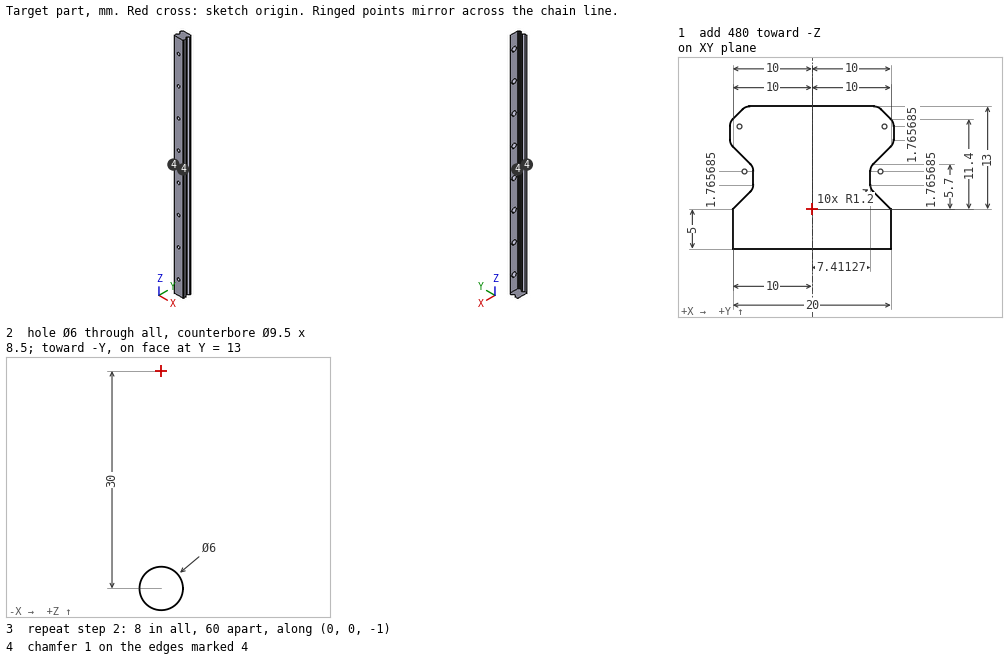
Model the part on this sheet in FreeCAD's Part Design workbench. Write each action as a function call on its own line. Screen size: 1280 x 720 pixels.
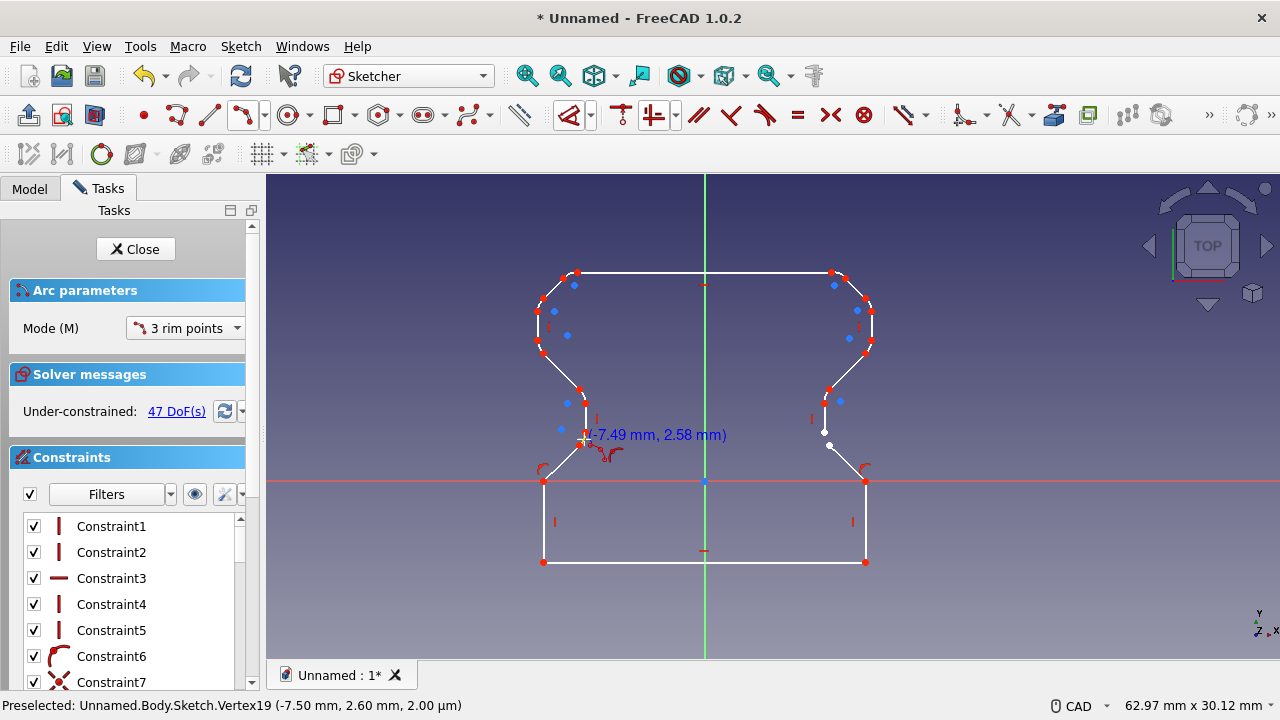
click(830, 446)
click(825, 433)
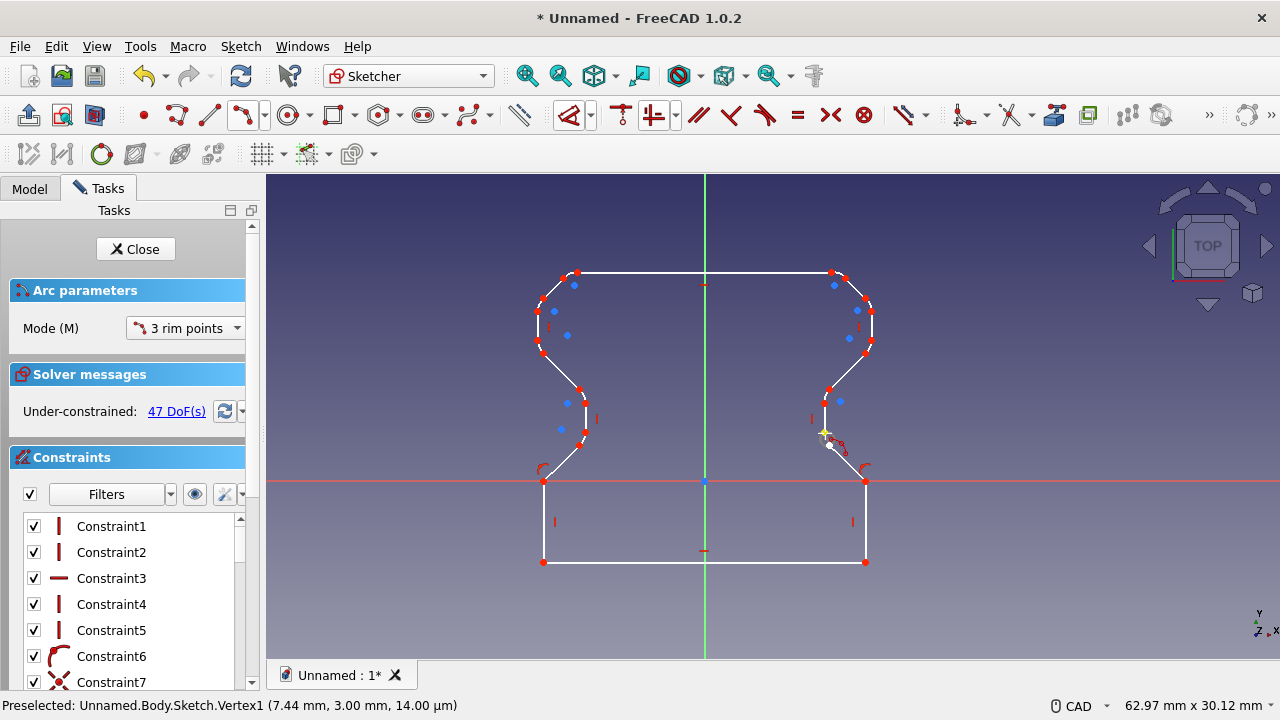
scroll(826, 439, up, 12)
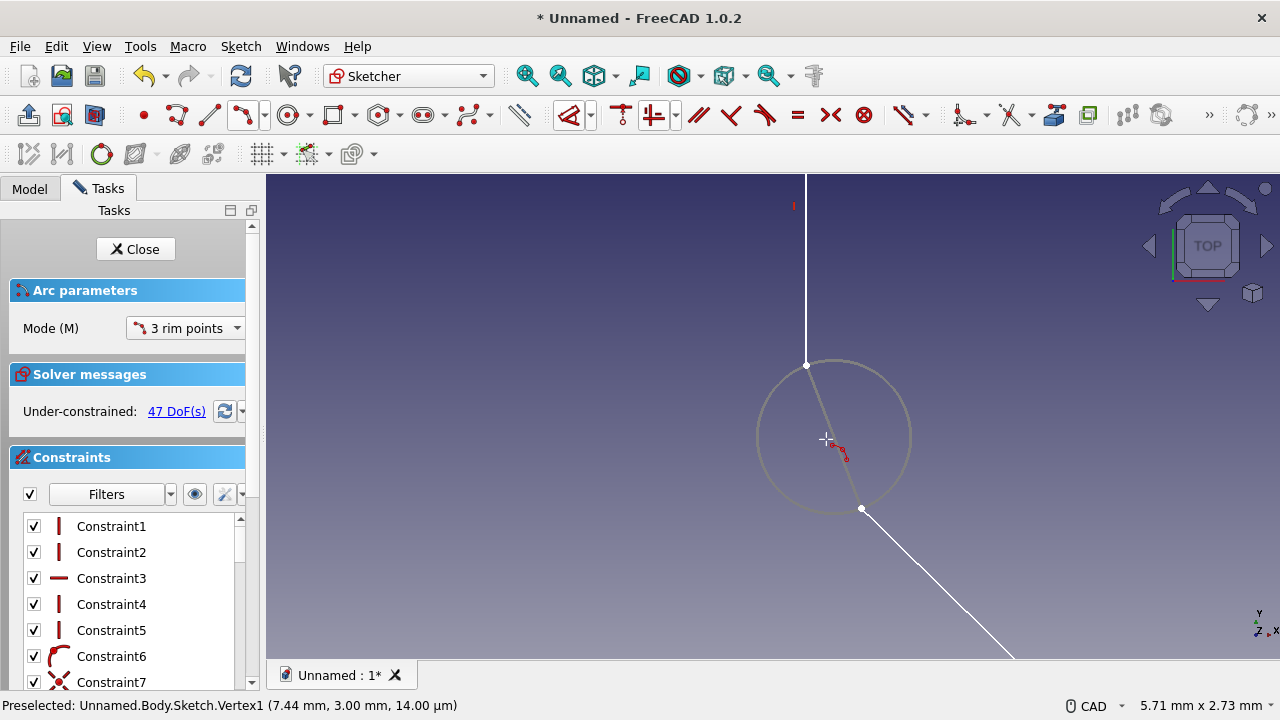
click(817, 431)
key(Escape)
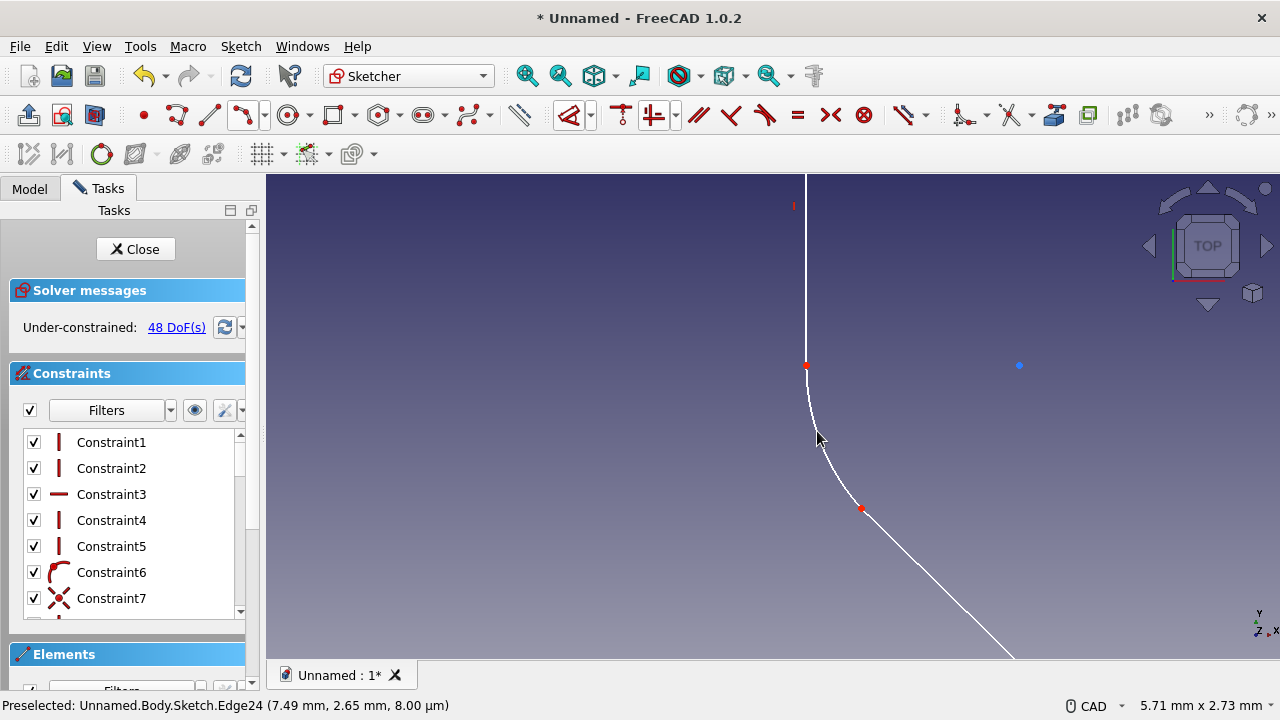
scroll(826, 439, down, 12)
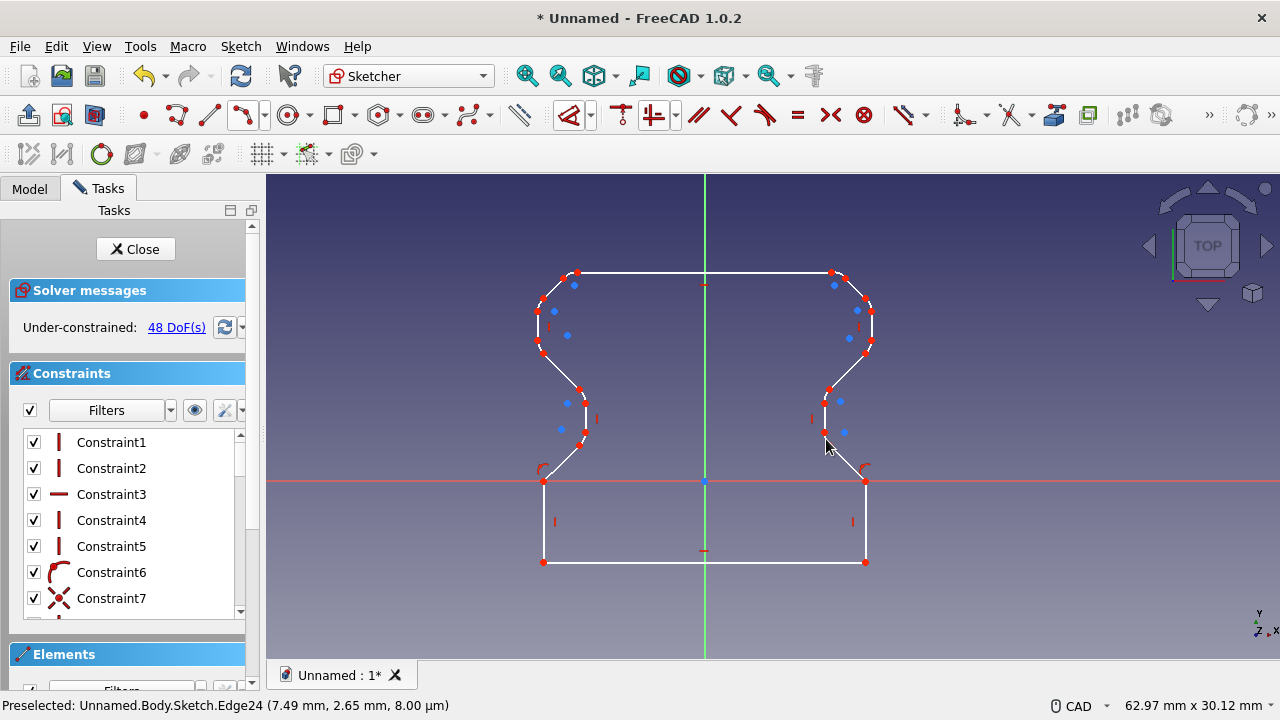
scroll(825, 424, up, 3)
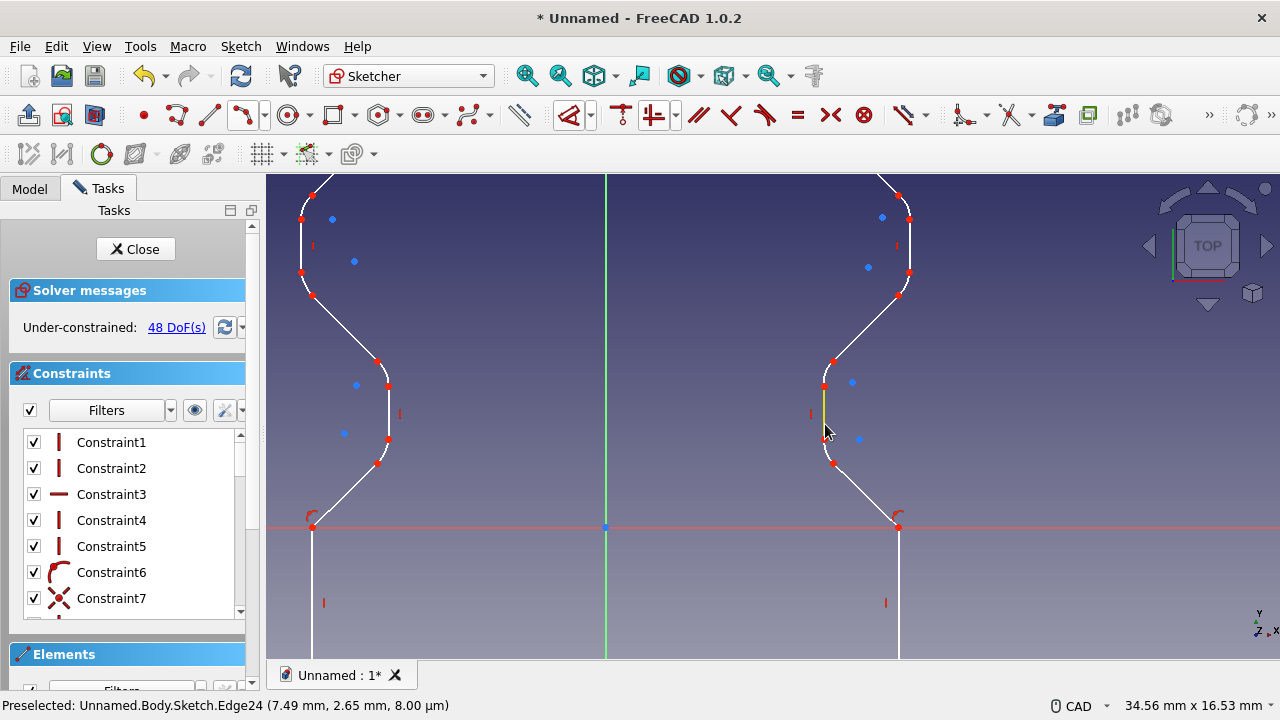
click(824, 424)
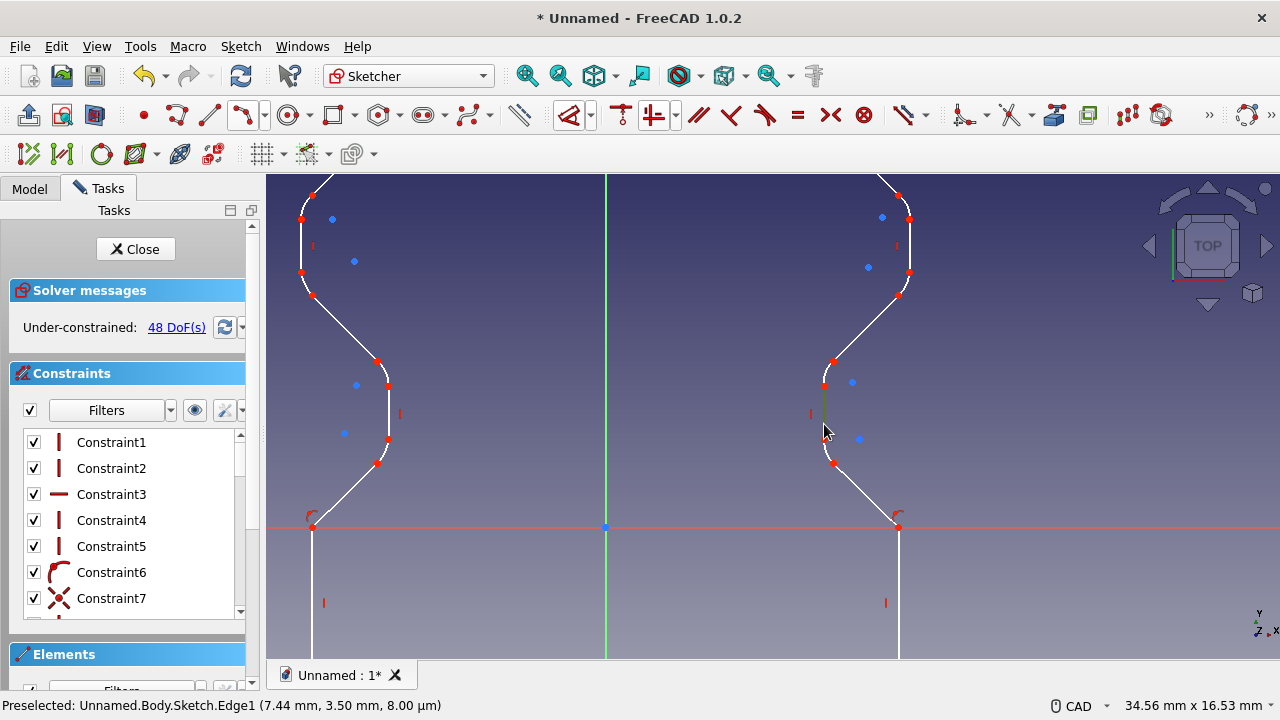
click(825, 373)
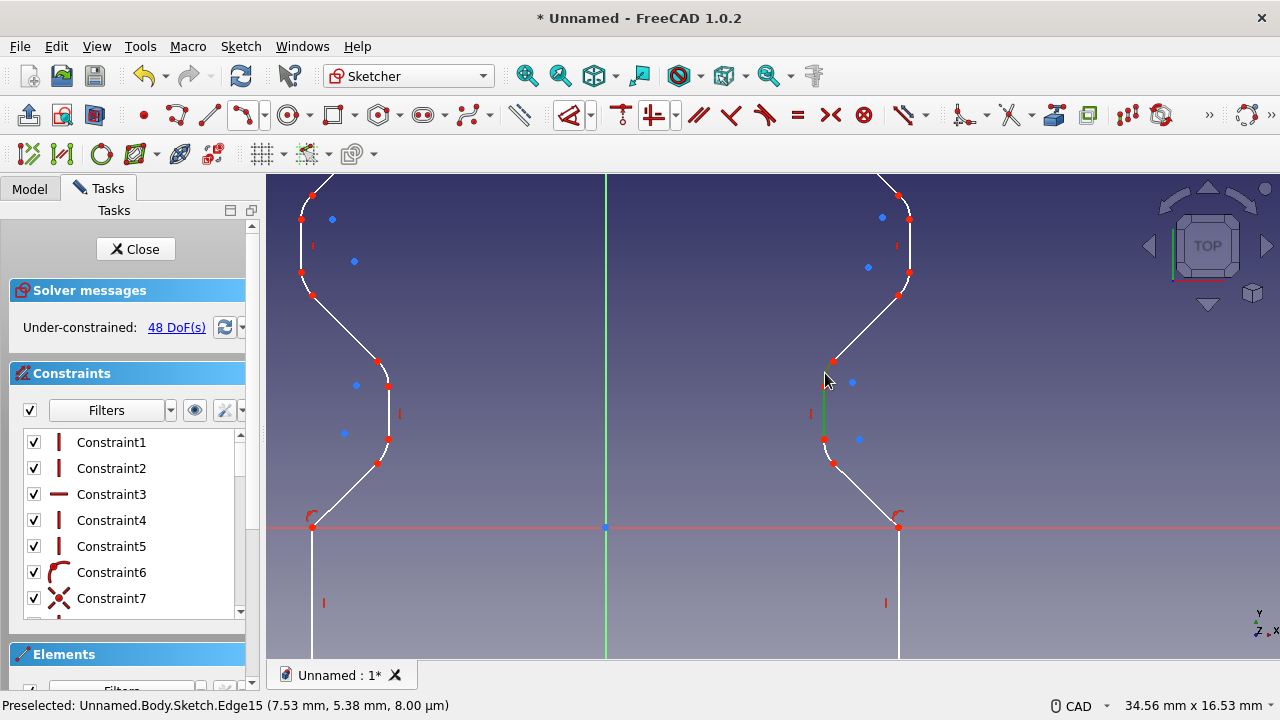
key(t)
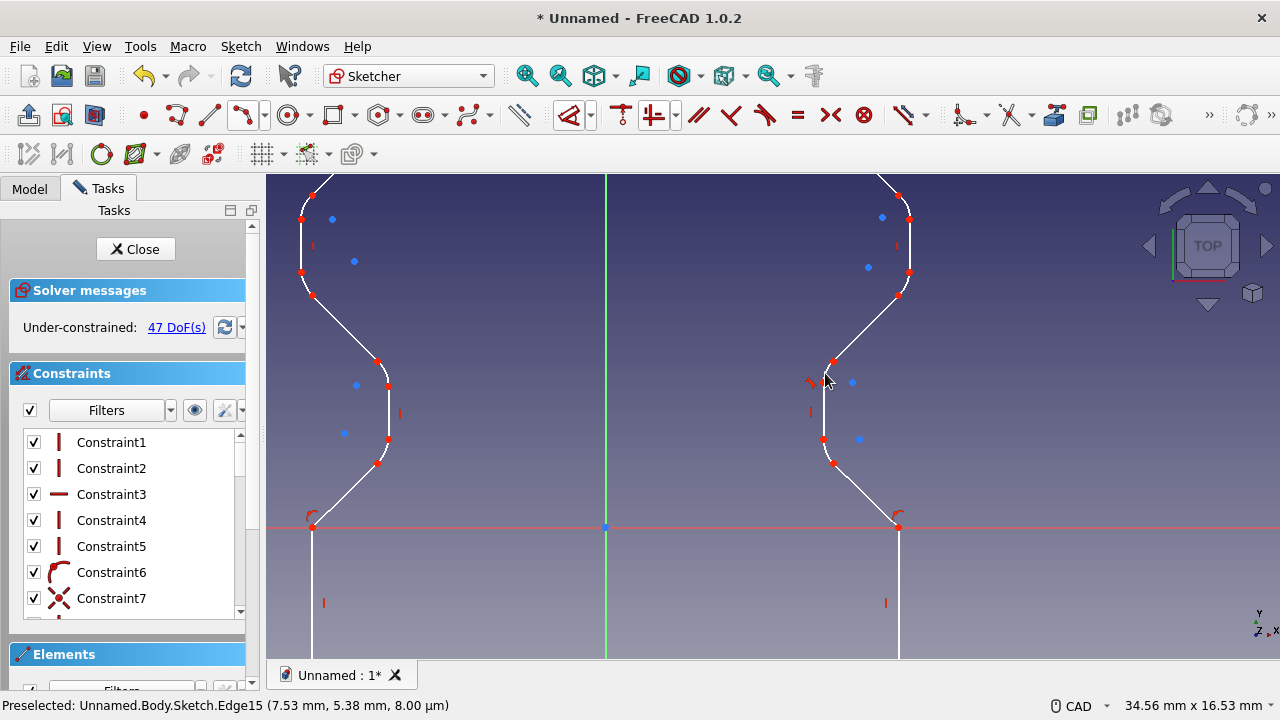
click(824, 423)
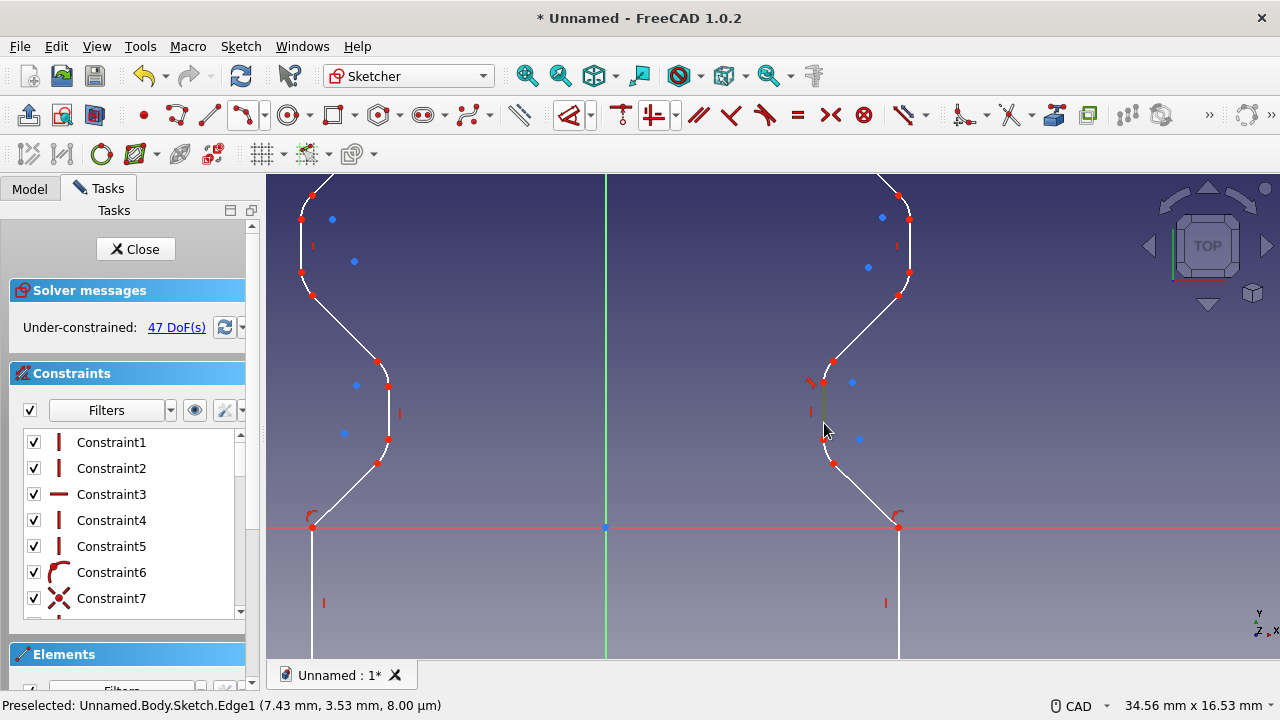
click(826, 452)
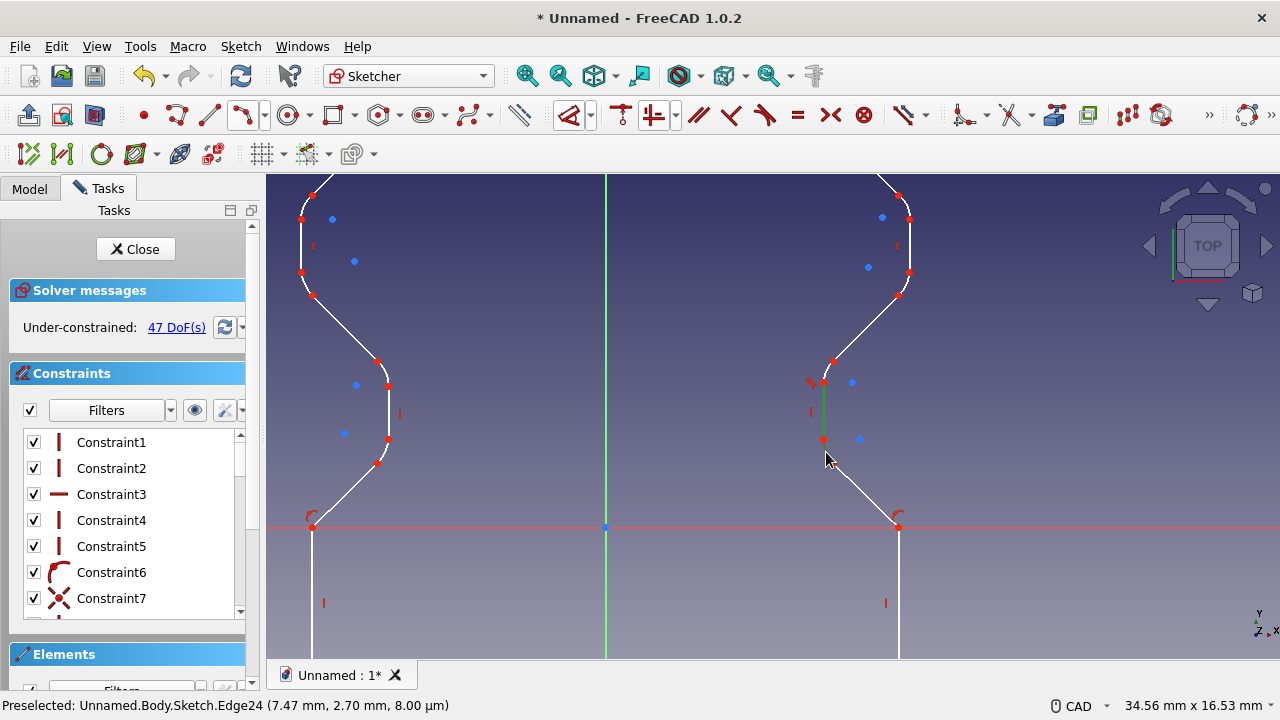
click(765, 116)